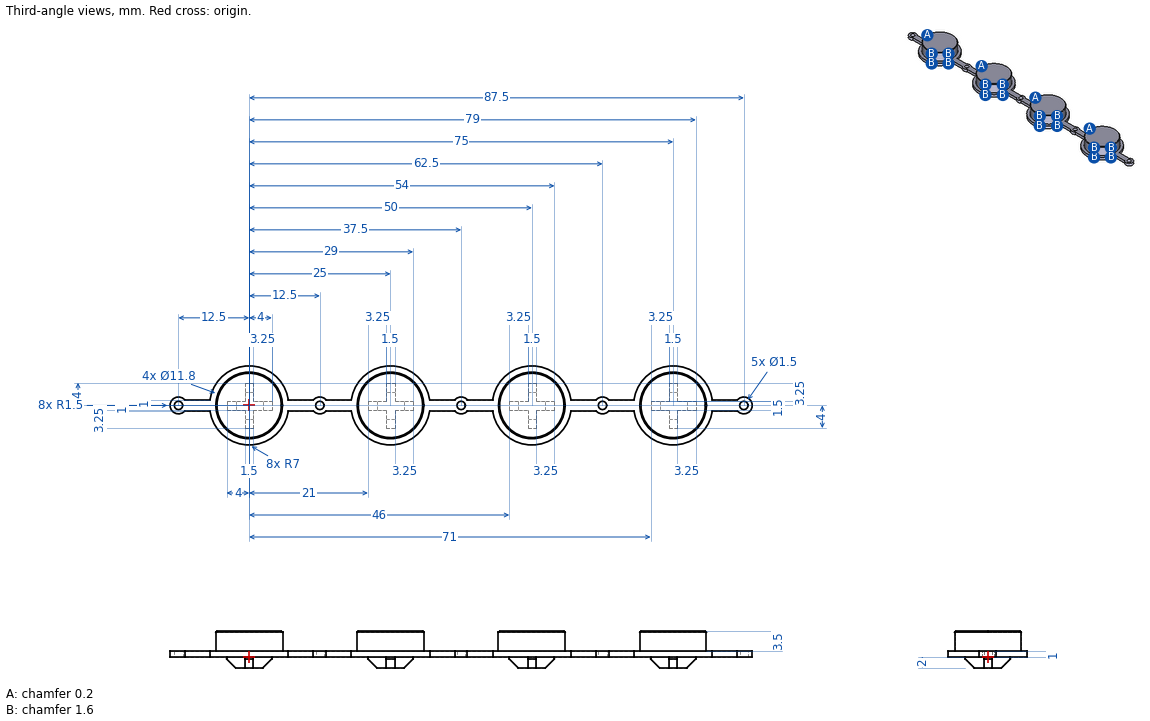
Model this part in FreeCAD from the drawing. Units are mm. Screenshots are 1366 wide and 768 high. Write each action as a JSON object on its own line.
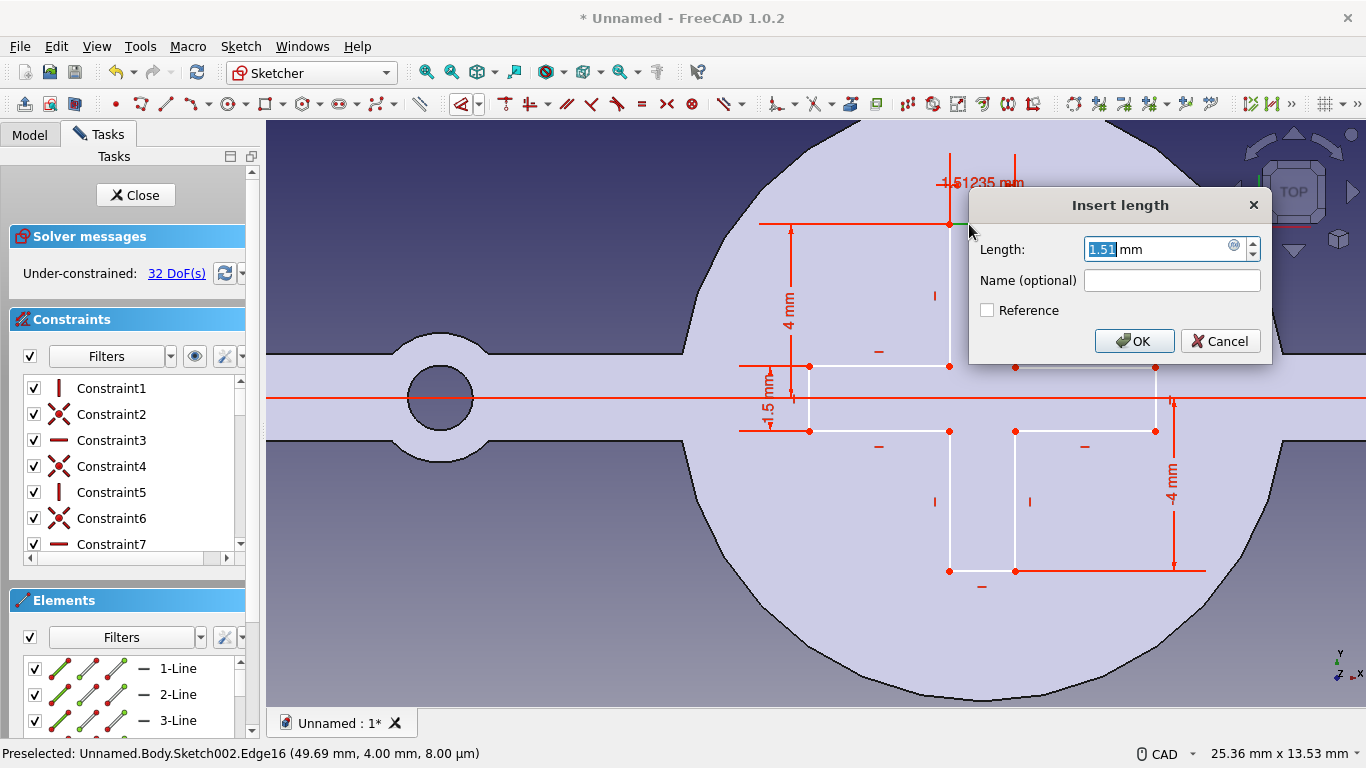
{"action": "type", "text": "1.5"}
{"action": "key", "text": "Return"}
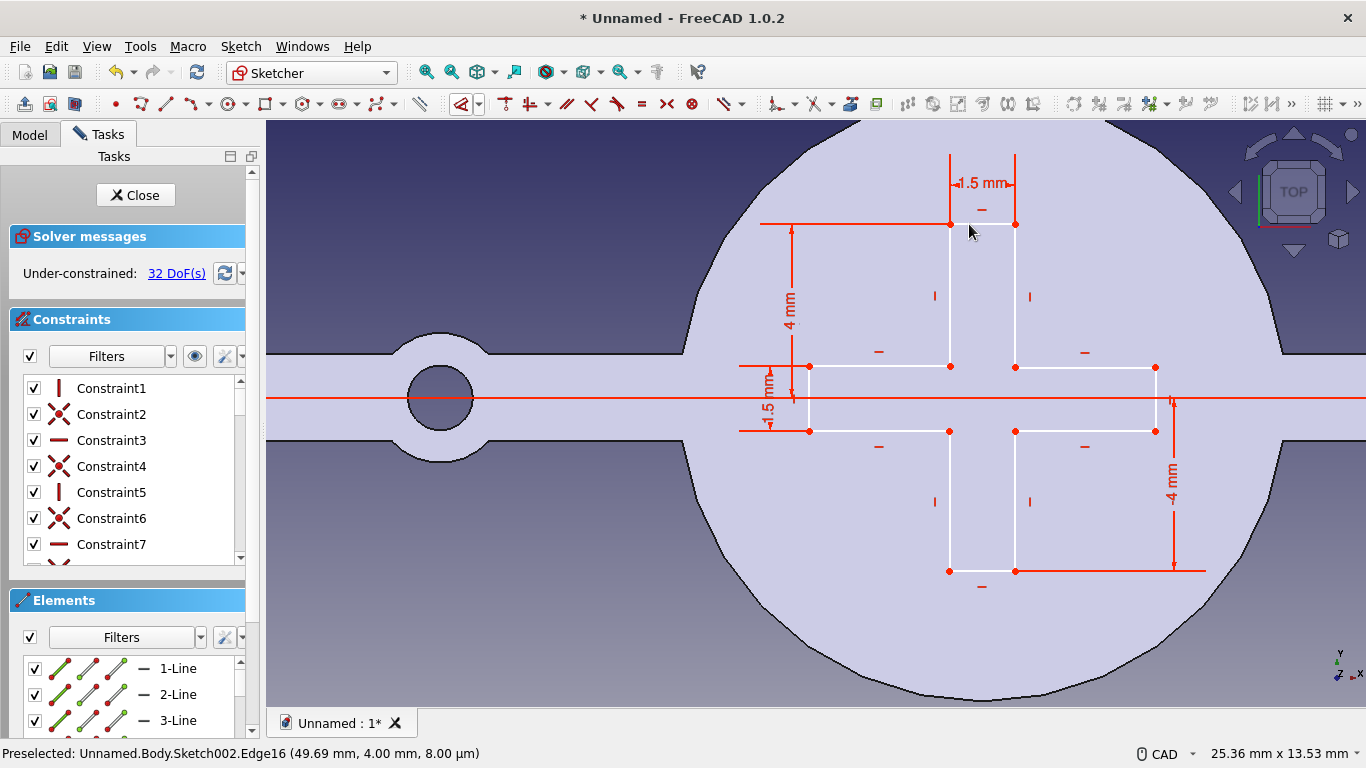
{"action": "scroll", "coordinate": [1156, 387], "scroll_direction": "up", "scroll_amount": 2}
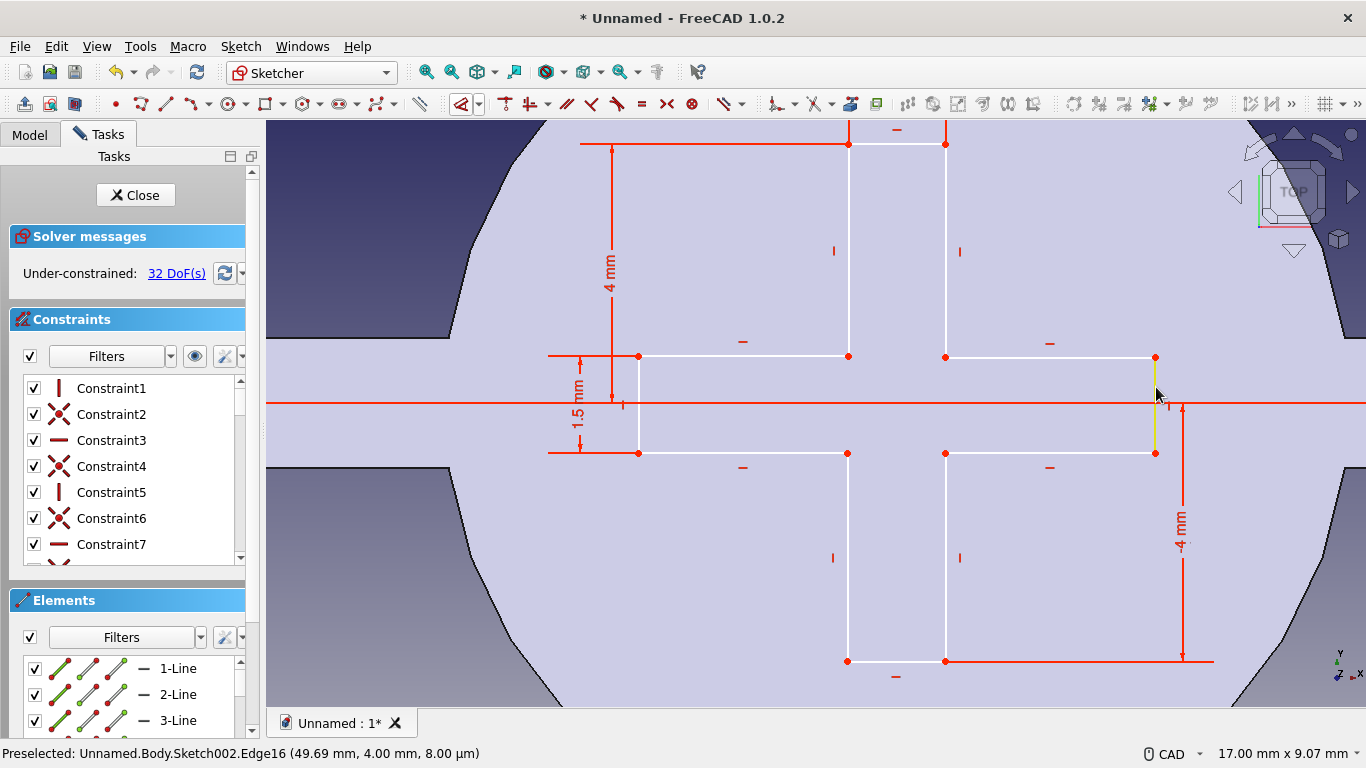
{"action": "left_click", "coordinate": [1155, 386]}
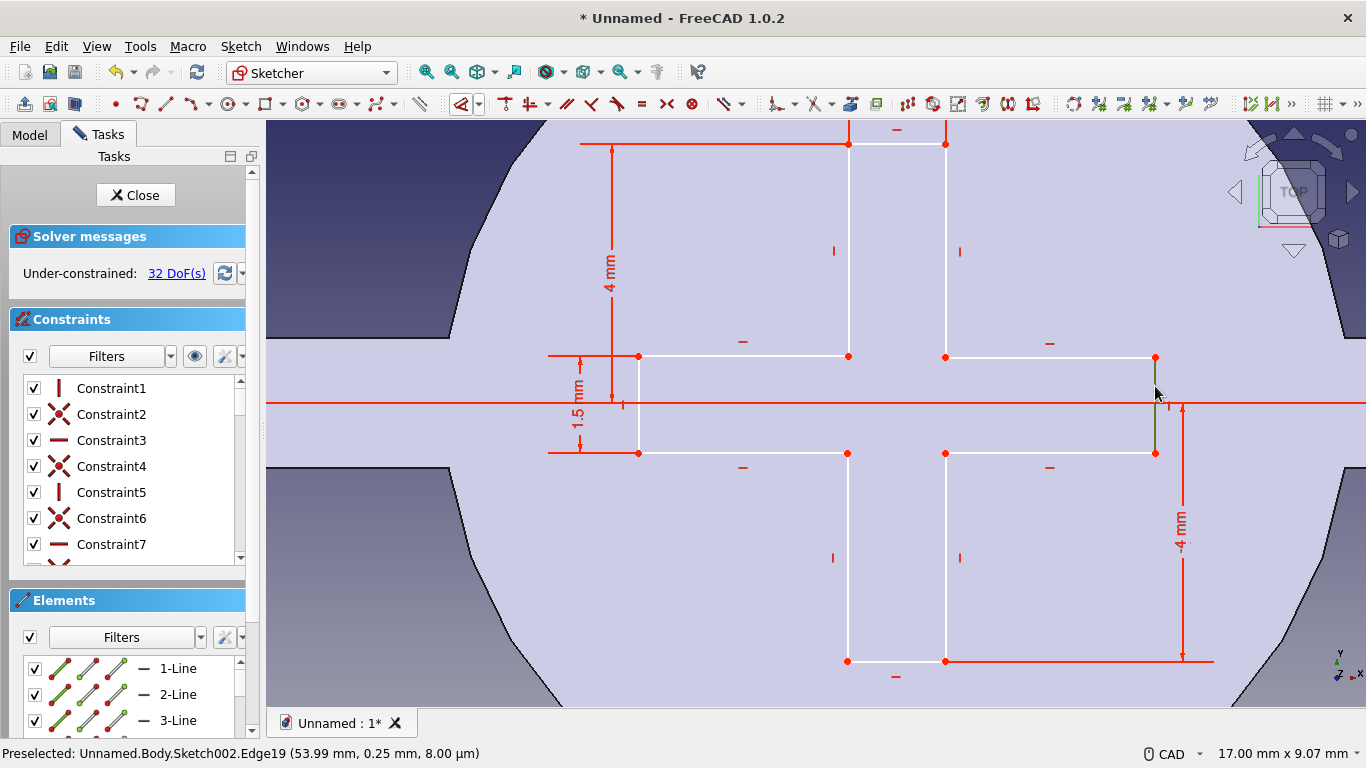
{"action": "key", "text": "i"}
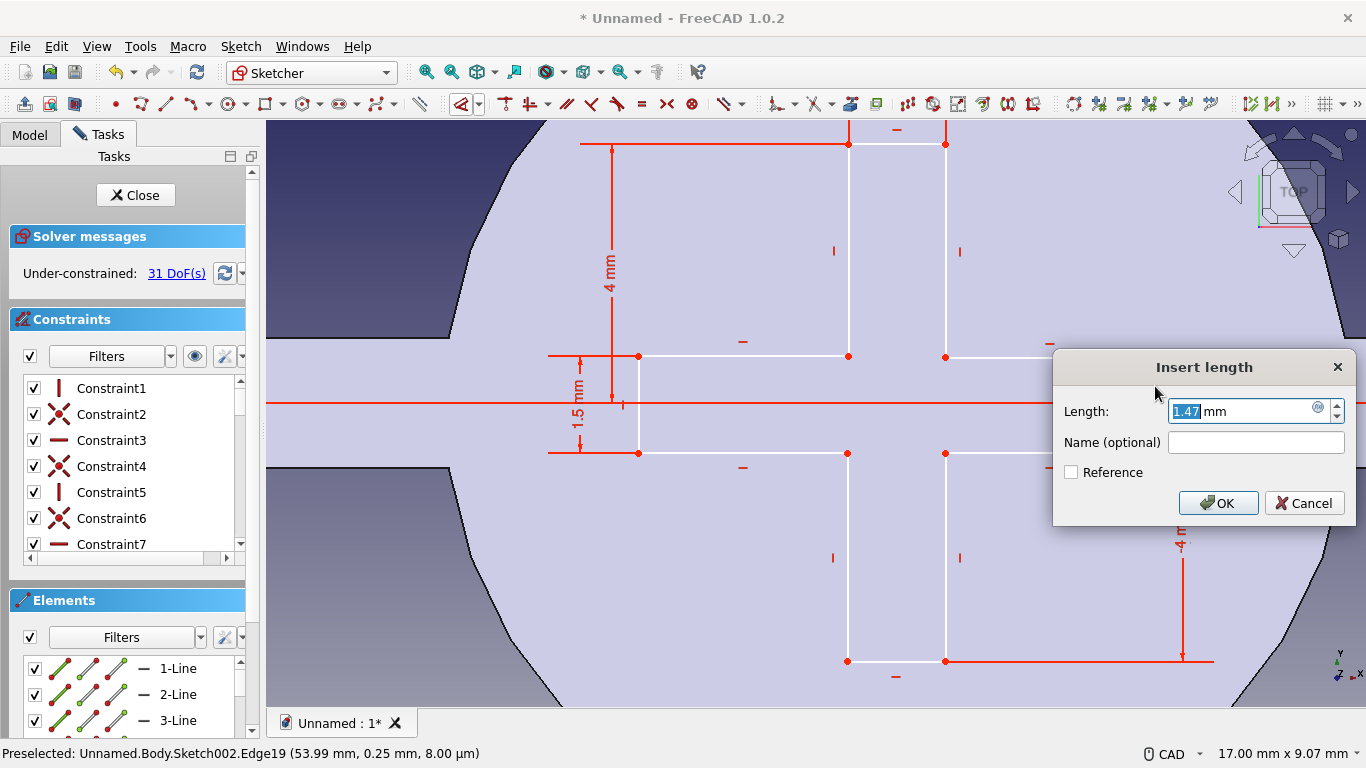
{"action": "type", "text": "1.5"}
{"action": "key", "text": "Return"}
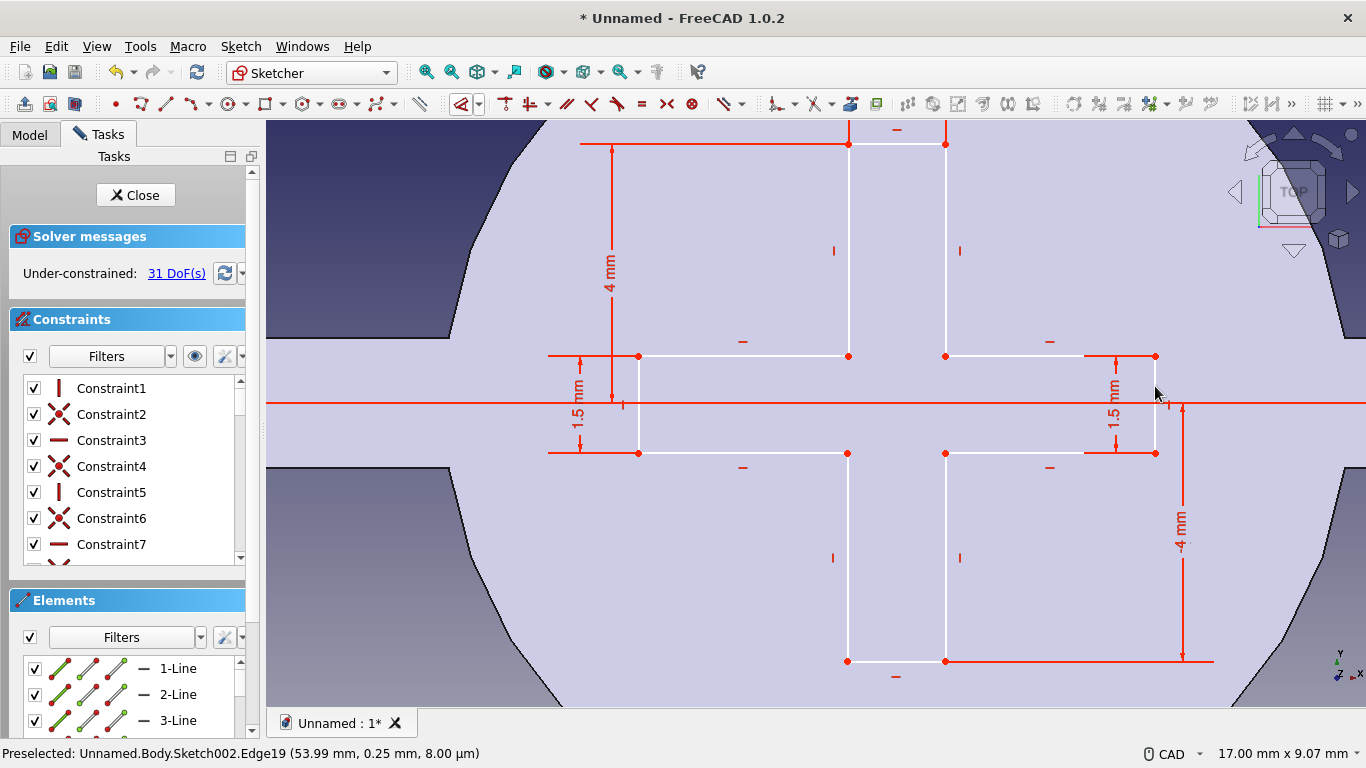
{"action": "left_click", "coordinate": [916, 662]}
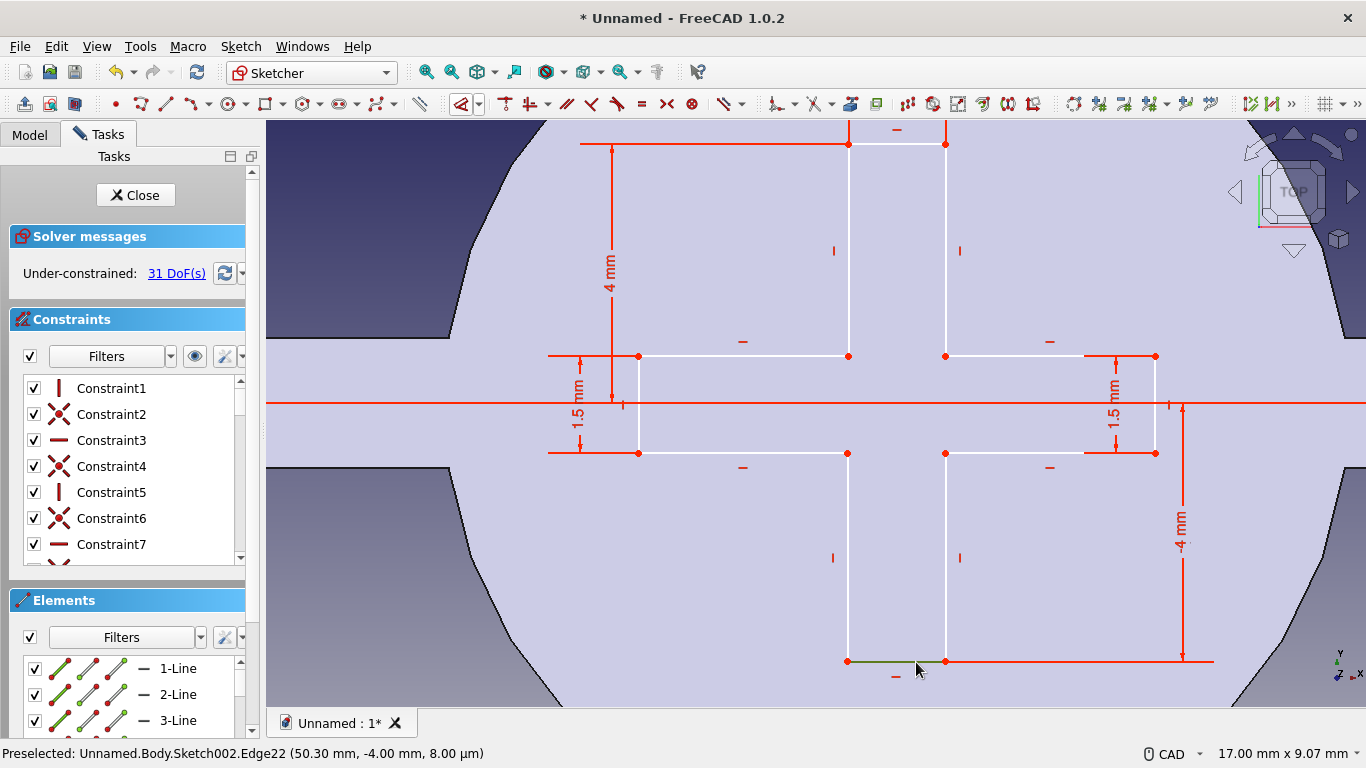
{"action": "key", "text": "l"}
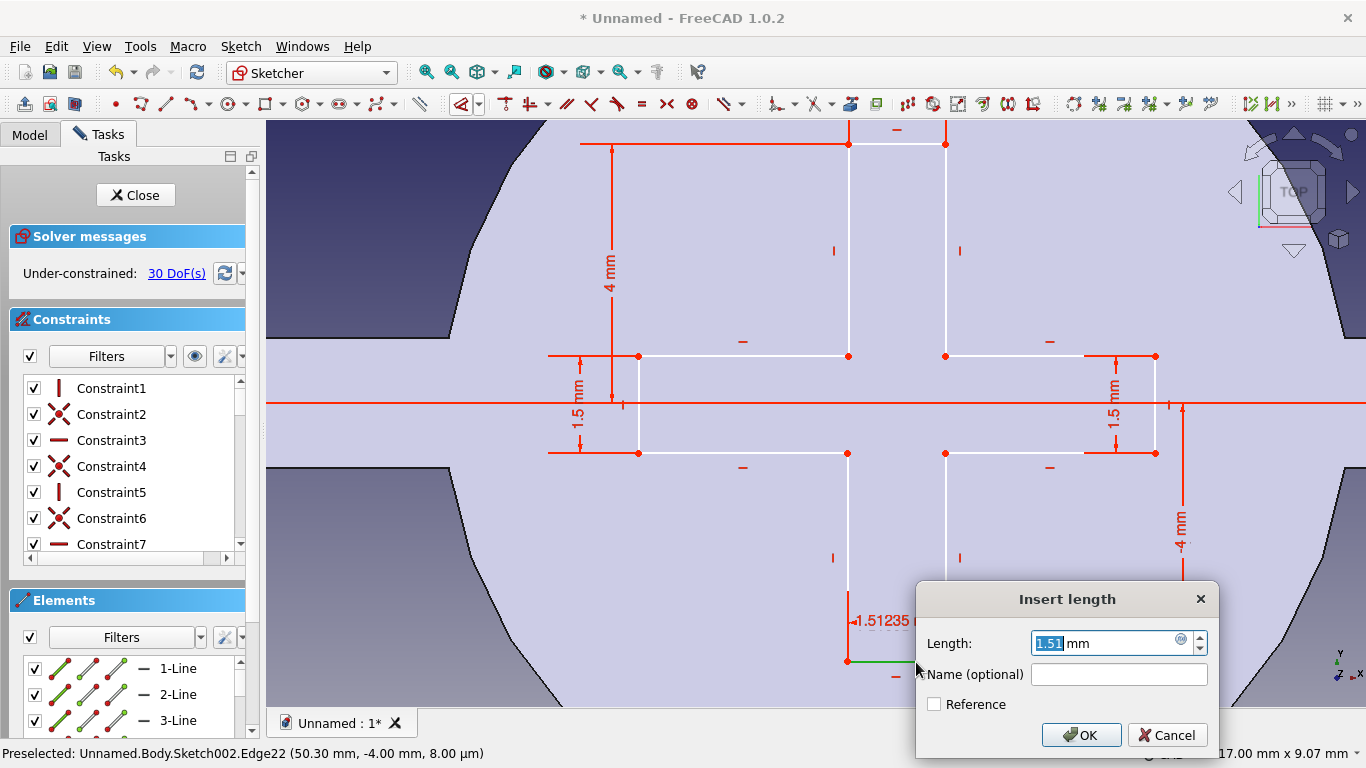
{"action": "type", "text": "1.5"}
{"action": "key", "text": "Return"}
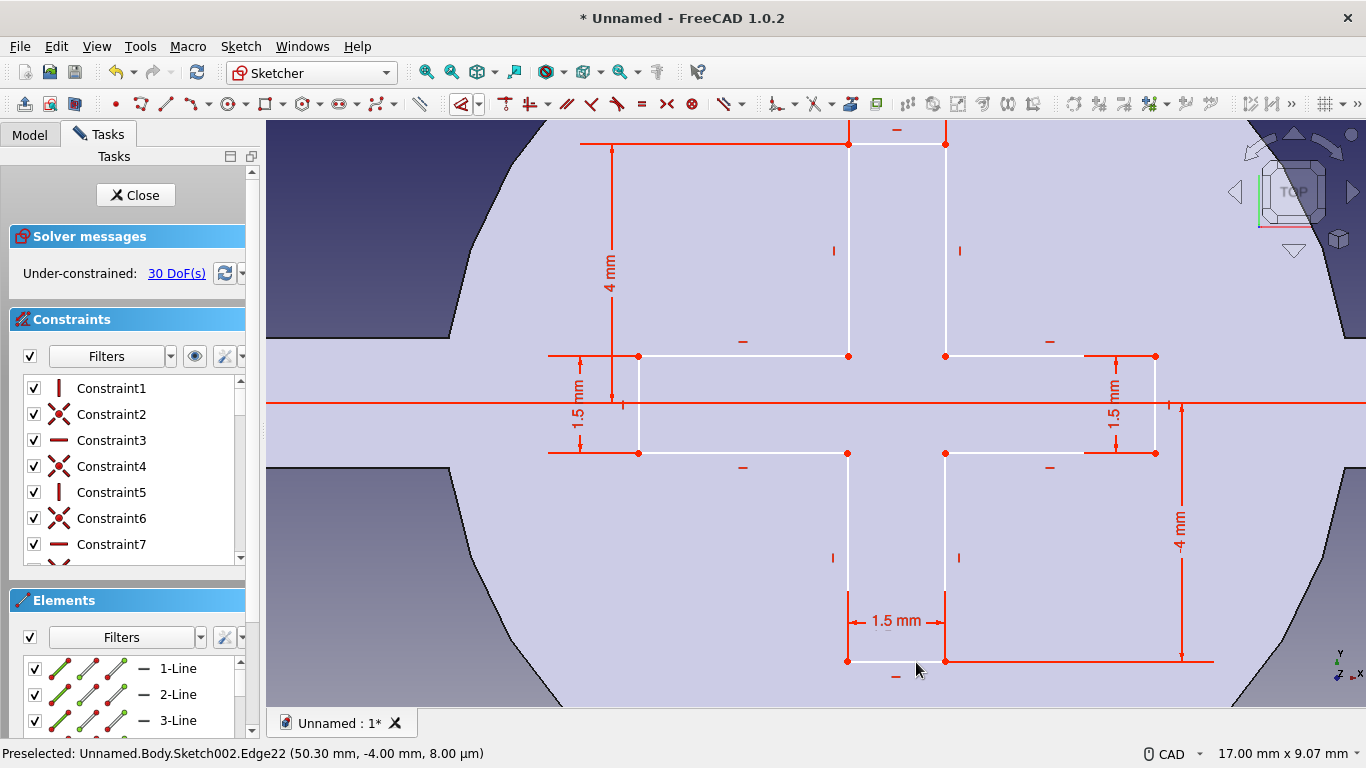
{"action": "scroll", "coordinate": [830, 415], "scroll_direction": "down", "scroll_amount": 11}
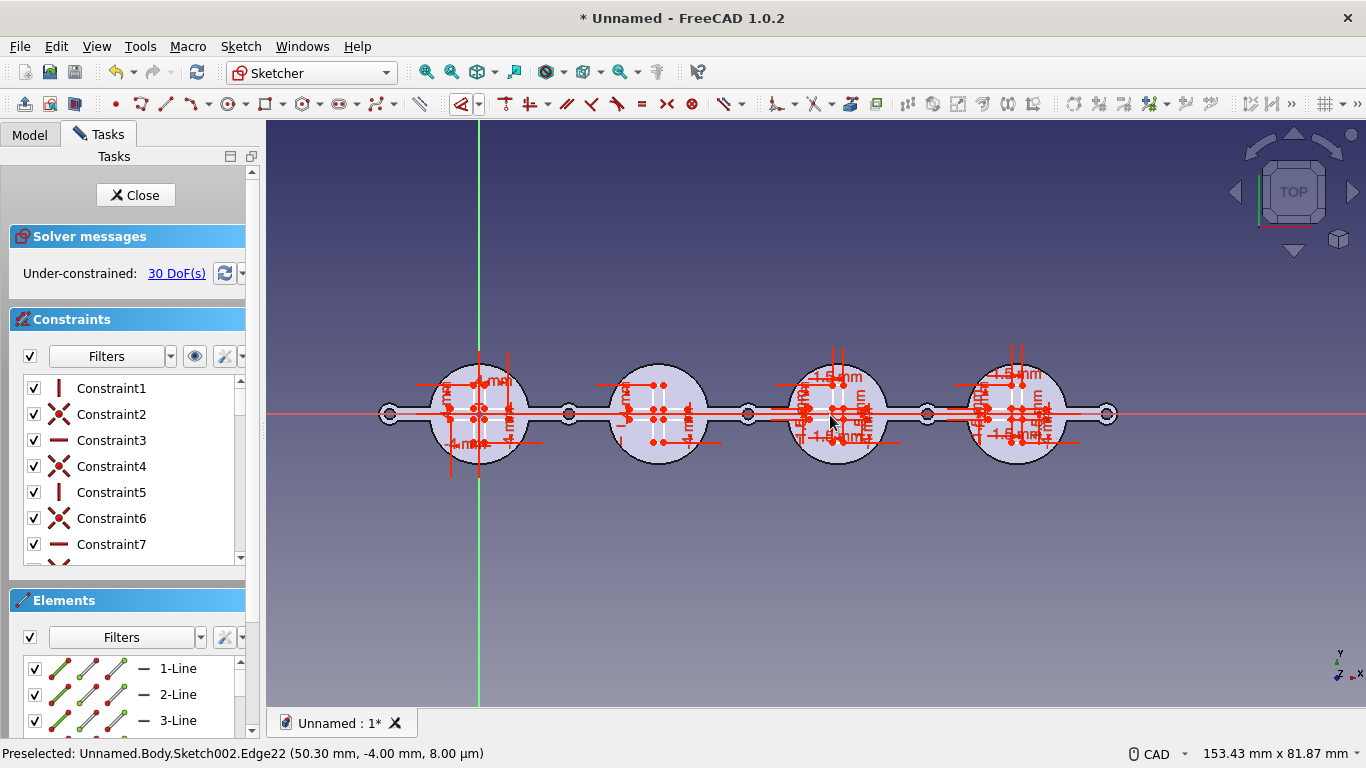
{"action": "scroll", "coordinate": [630, 417], "scroll_direction": "up", "scroll_amount": 9}